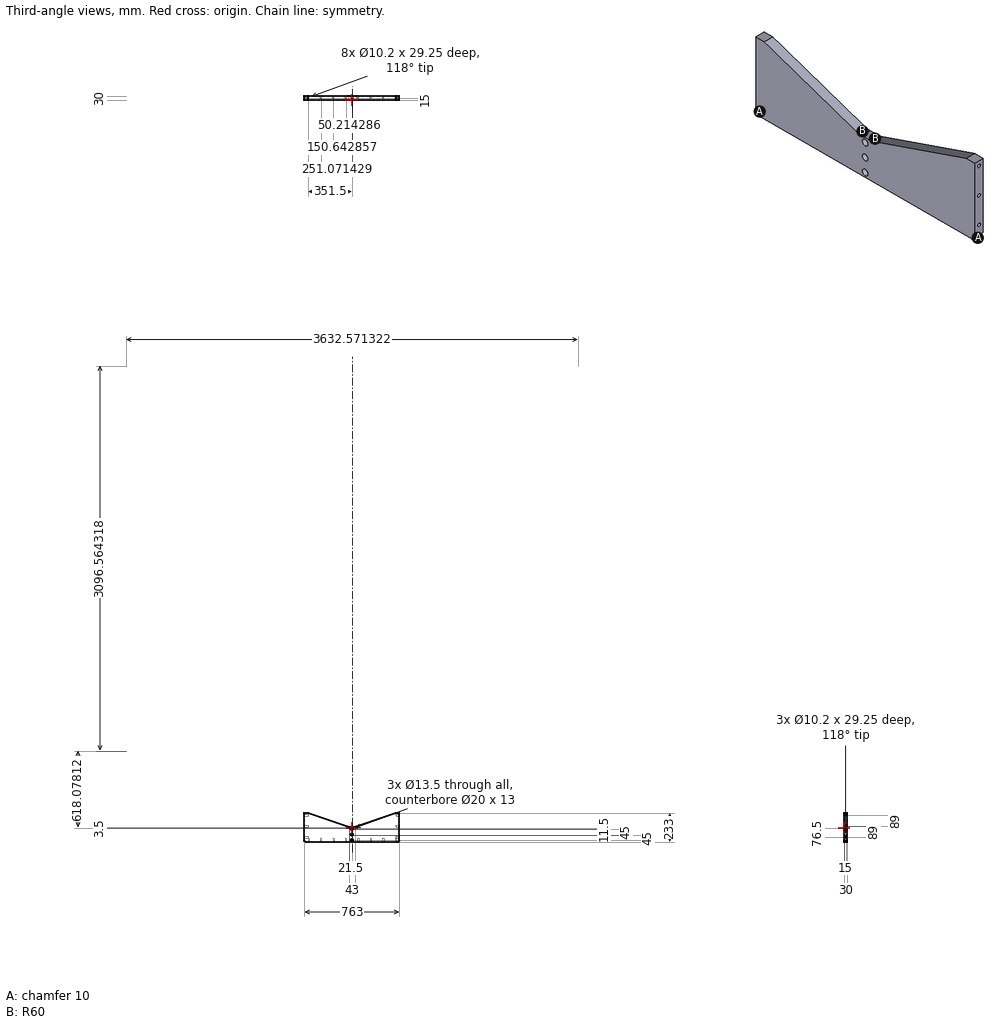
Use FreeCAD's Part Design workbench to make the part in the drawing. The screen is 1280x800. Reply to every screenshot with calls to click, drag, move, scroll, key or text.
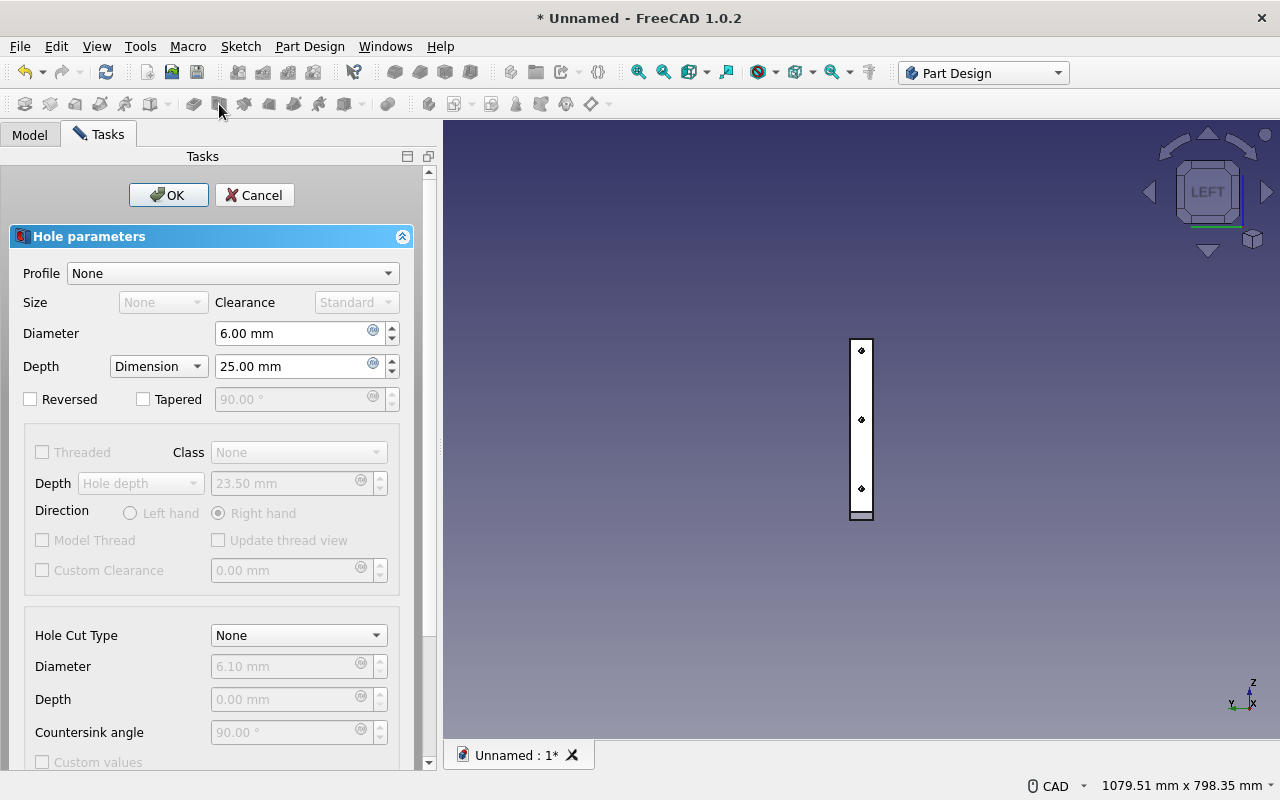
triple_click(300, 334)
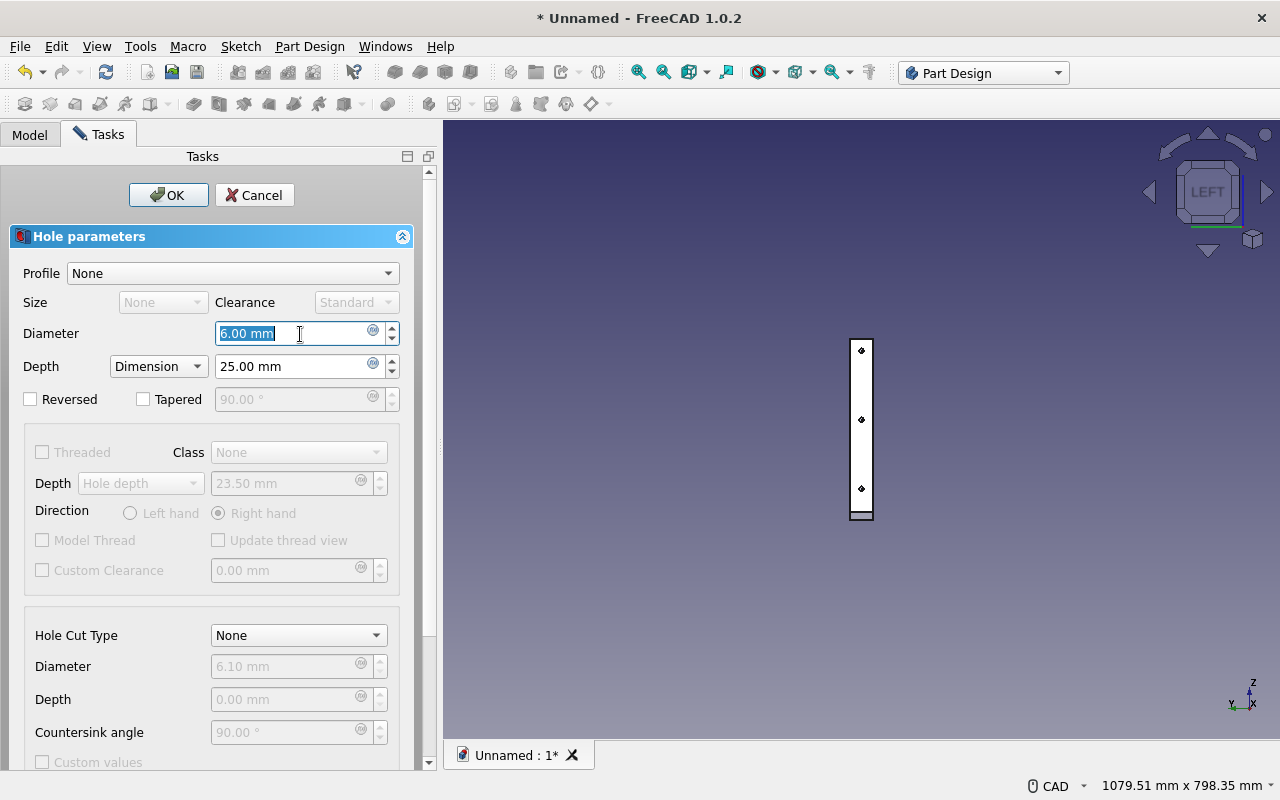
text(10.2)
key(Tab)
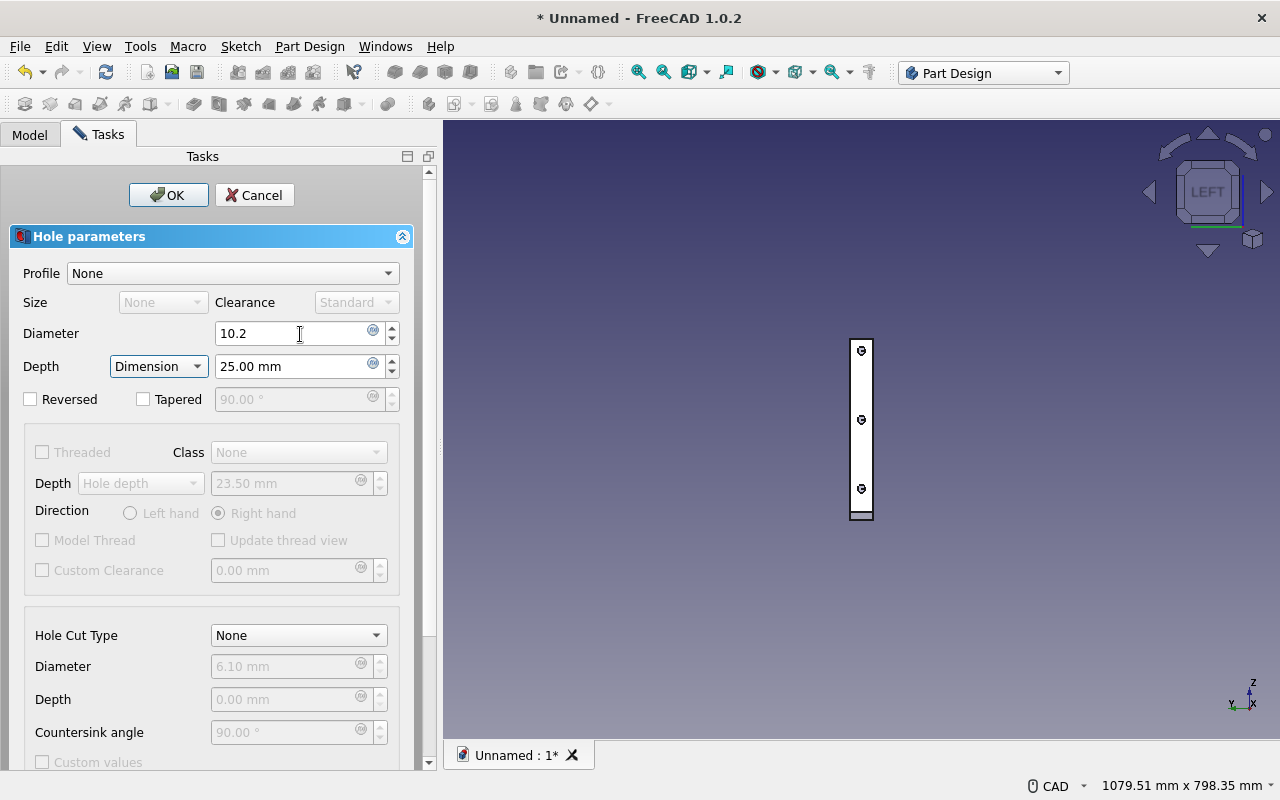
triple_click(300, 366)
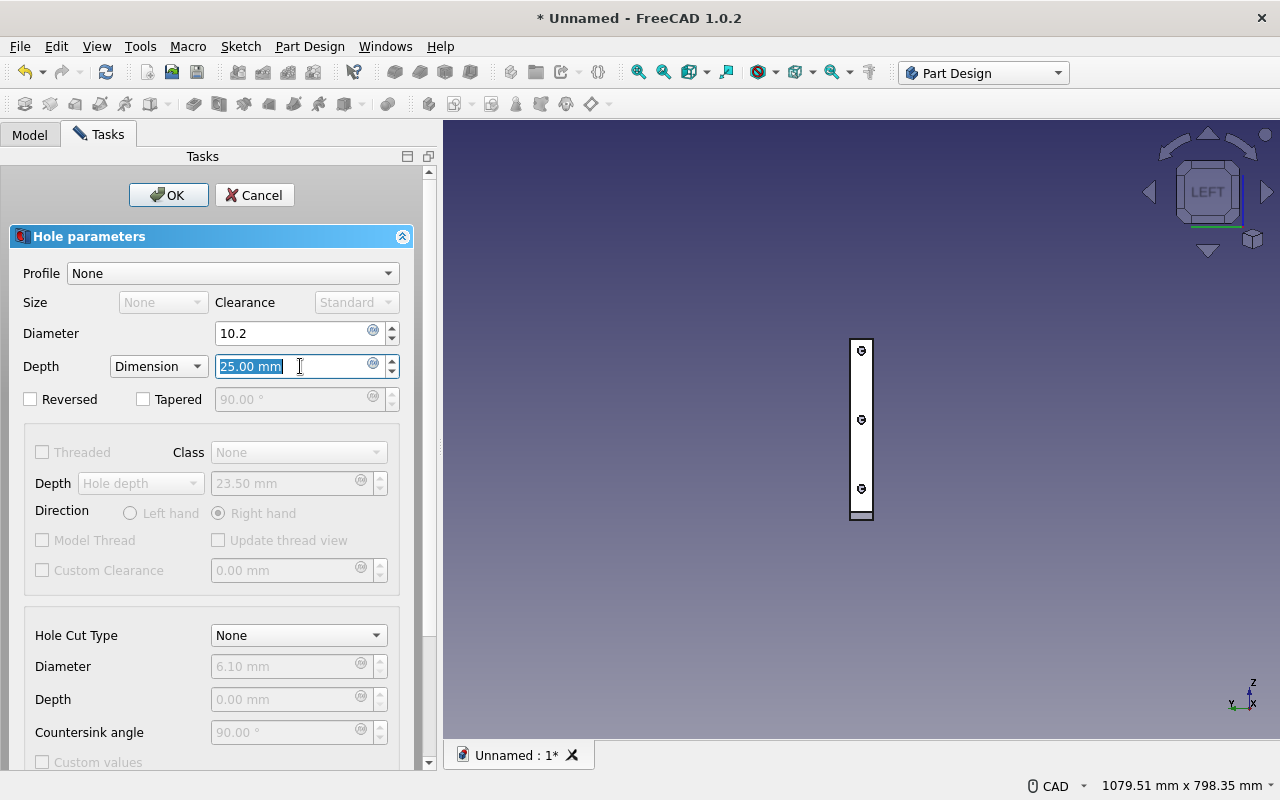
text(29.25)
key(Tab)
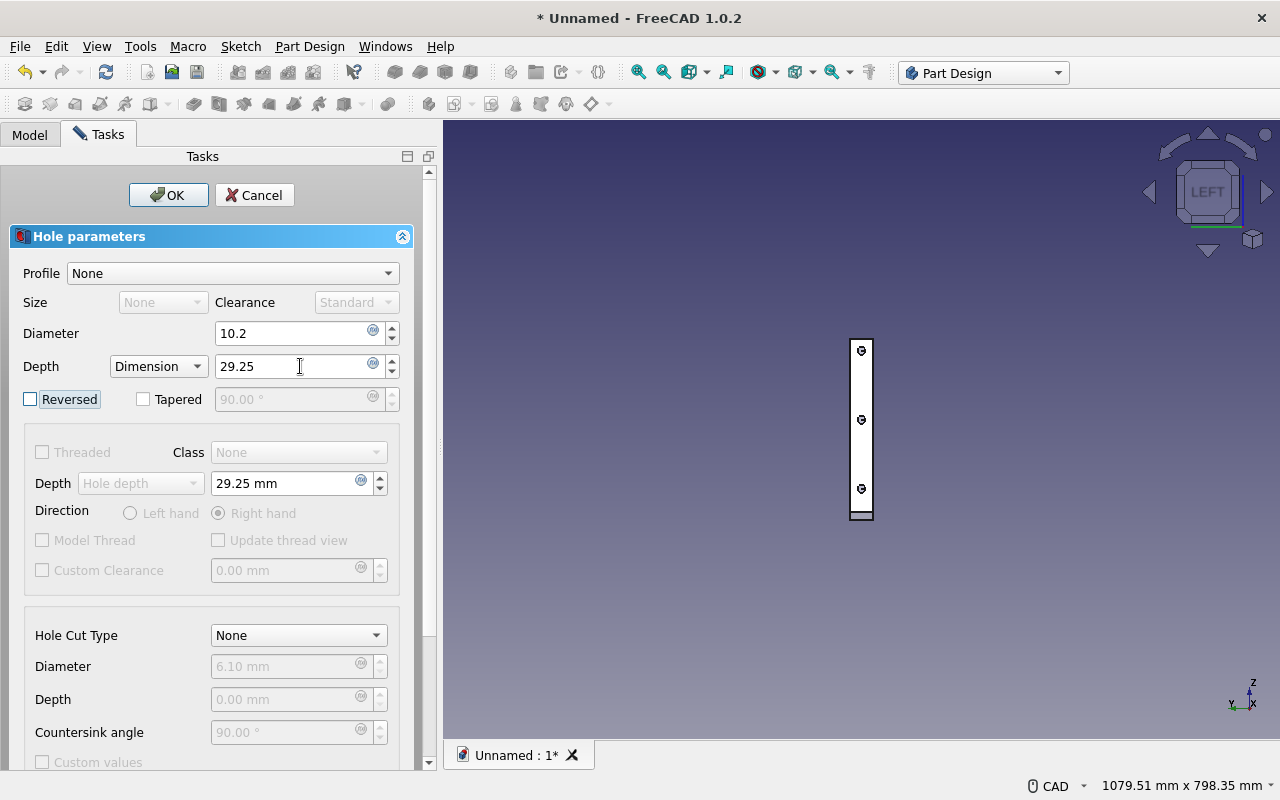
click(169, 195)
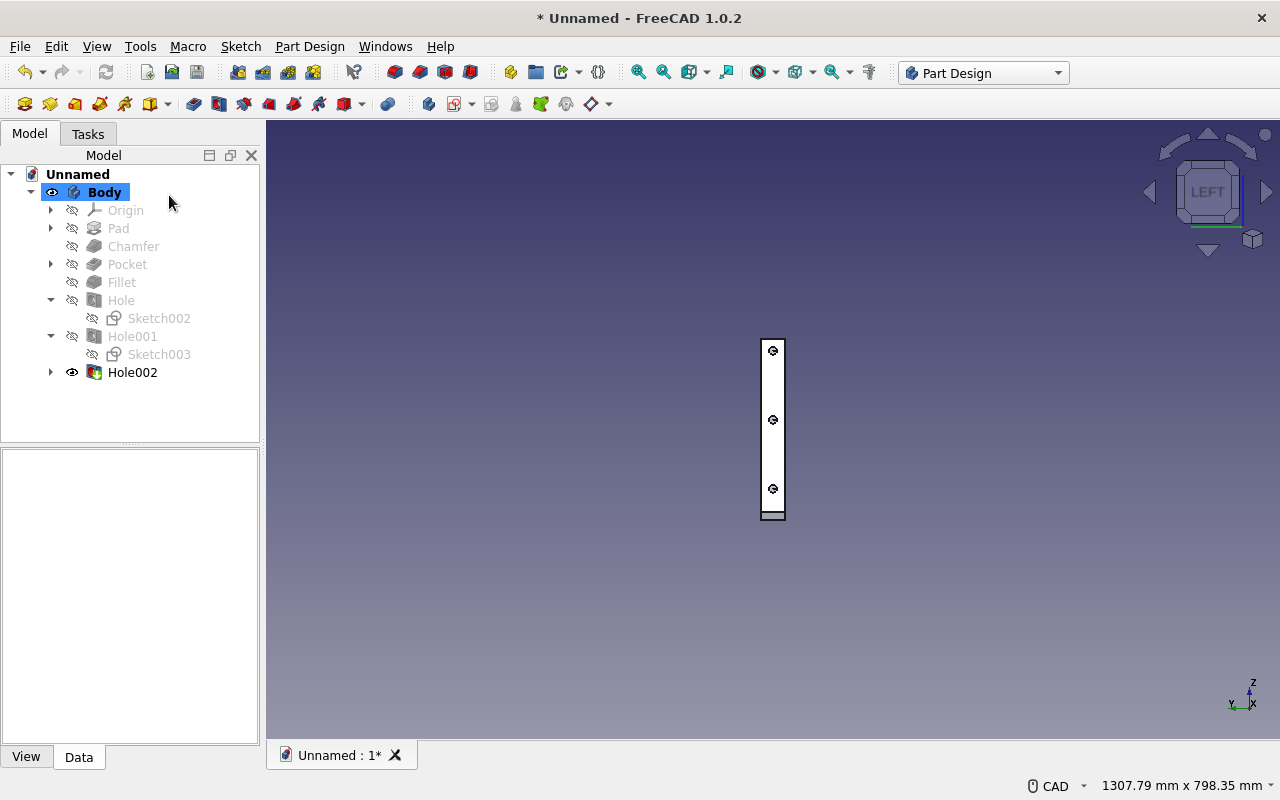
key(v)
key(f)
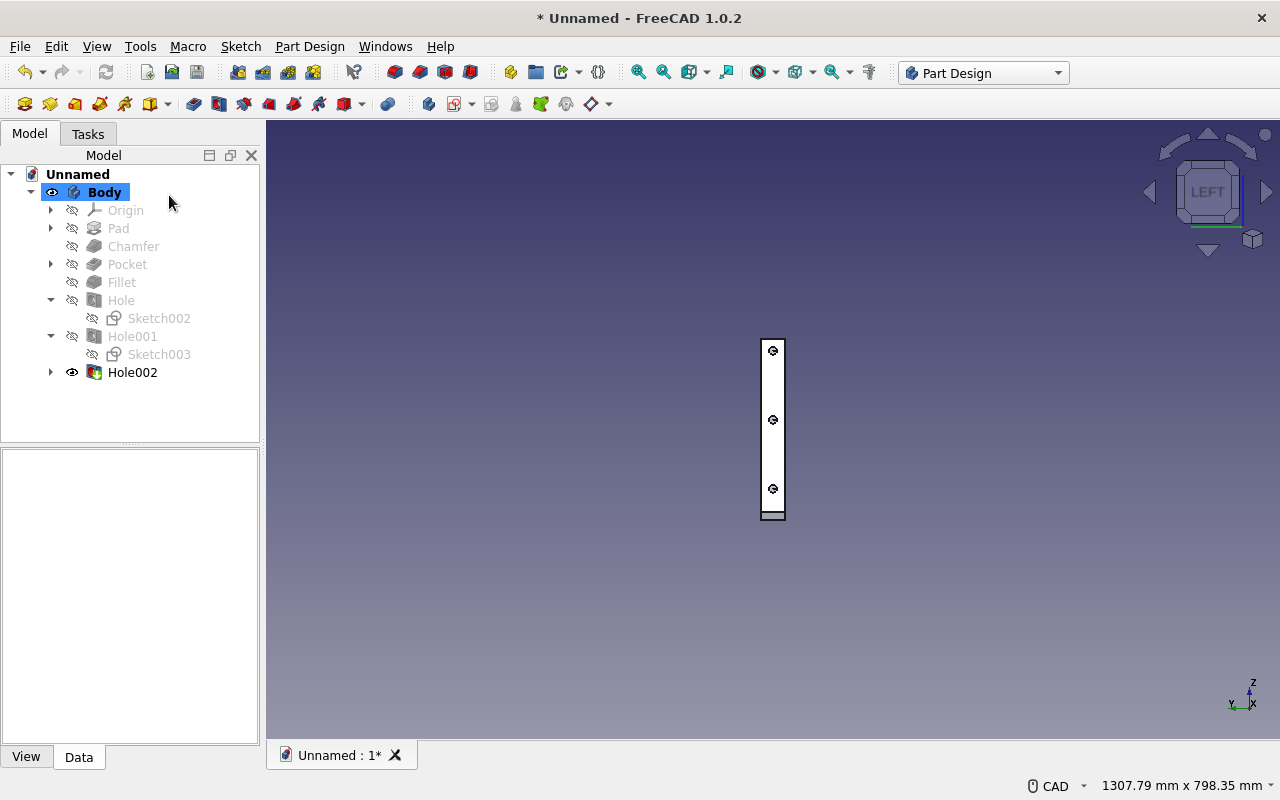
key(0)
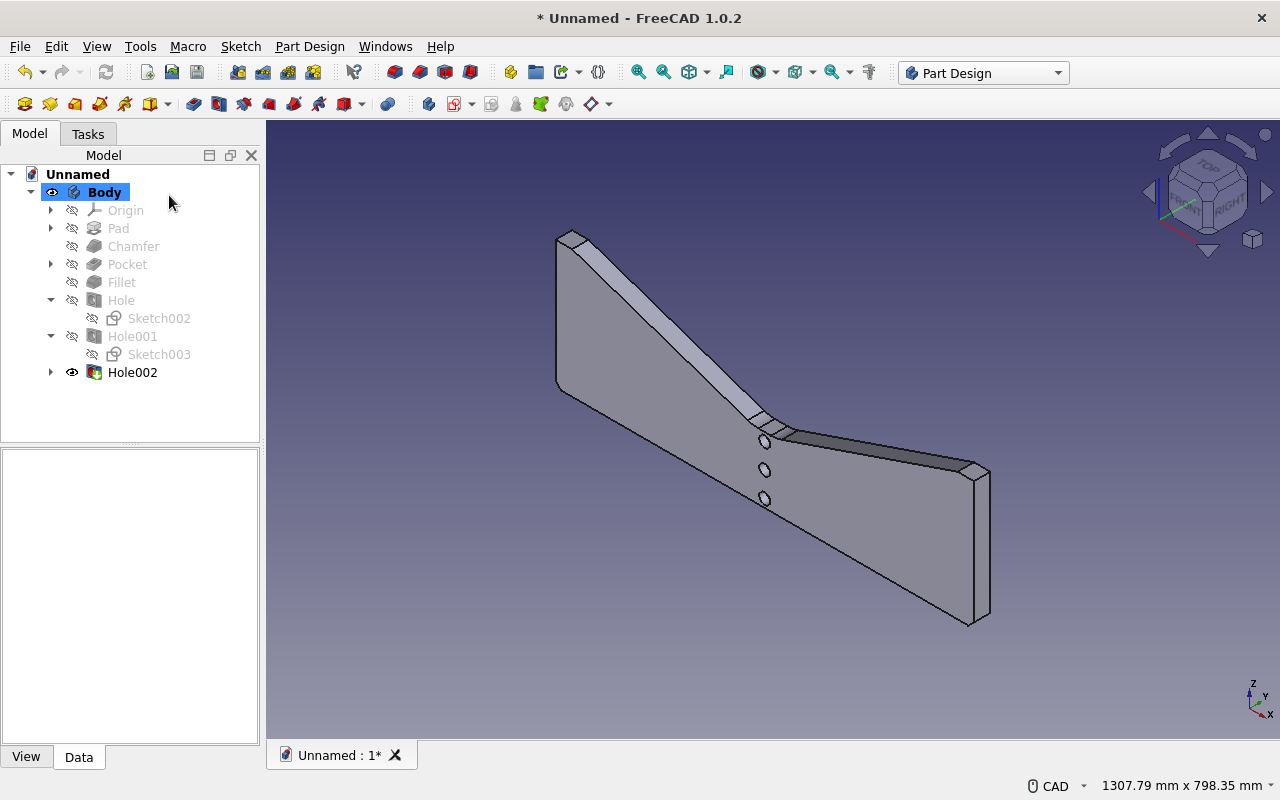
click(982, 506)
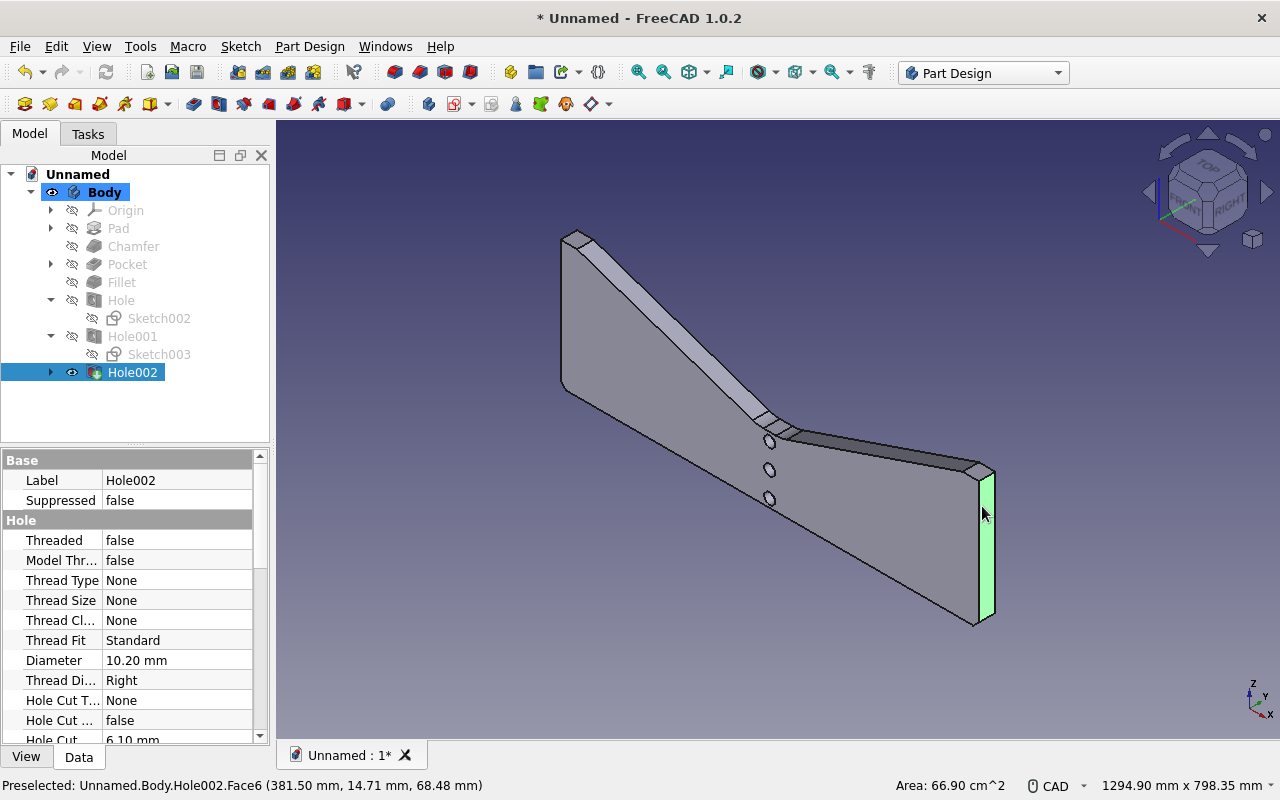
click(454, 104)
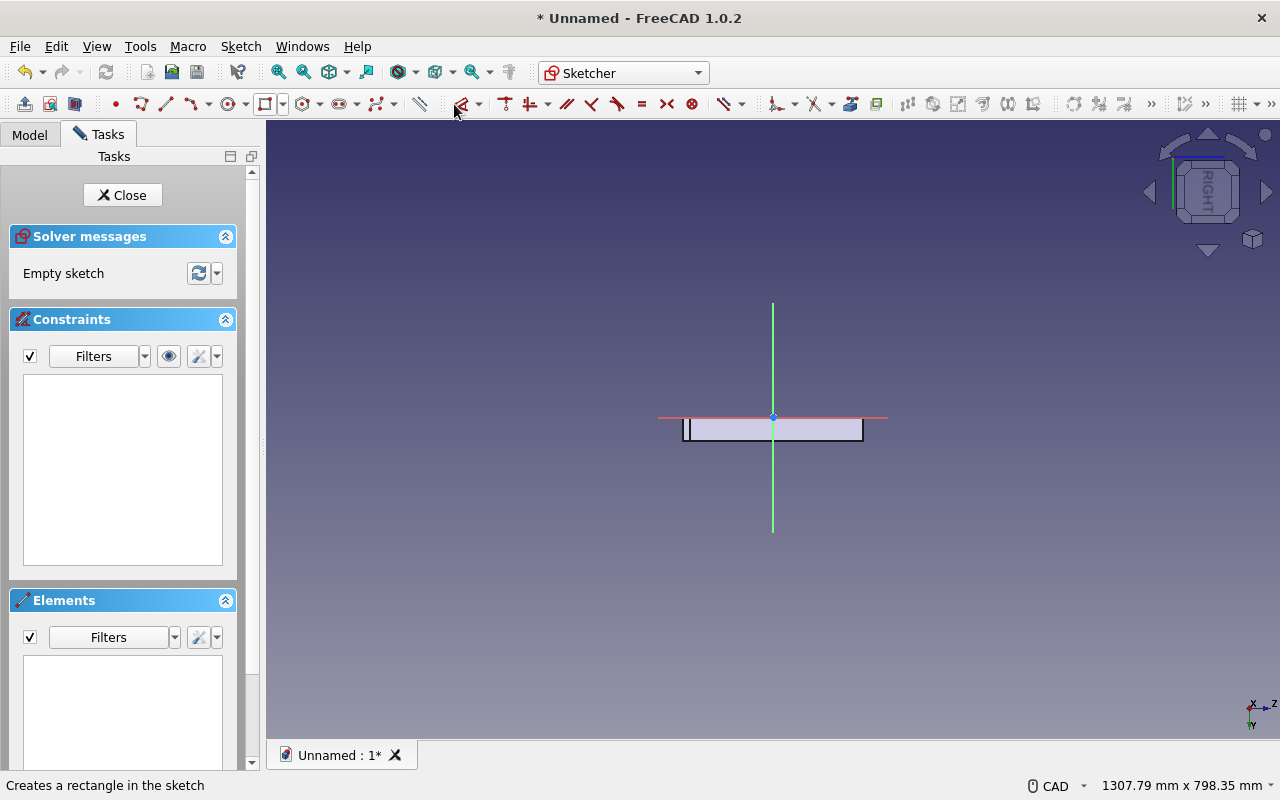
scroll(808, 424, up, 7)